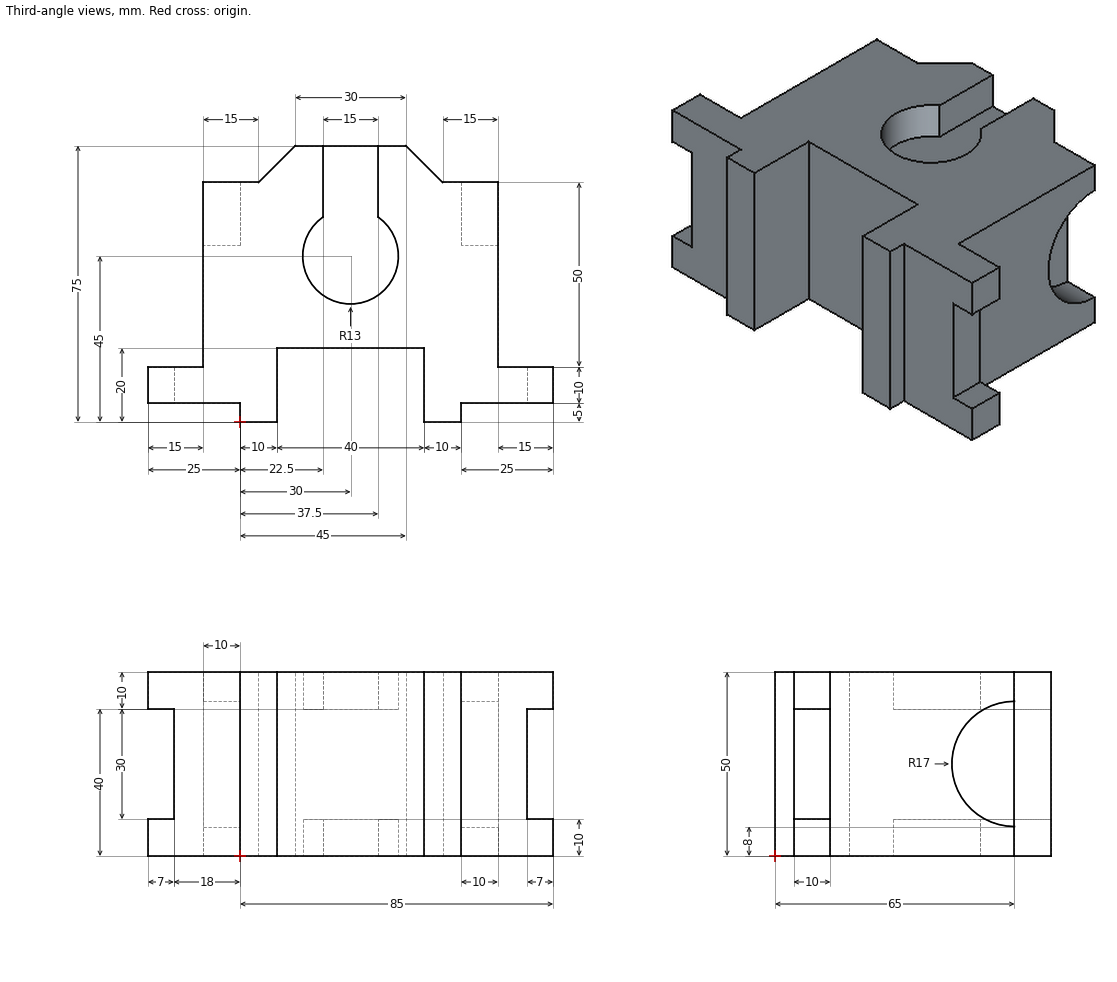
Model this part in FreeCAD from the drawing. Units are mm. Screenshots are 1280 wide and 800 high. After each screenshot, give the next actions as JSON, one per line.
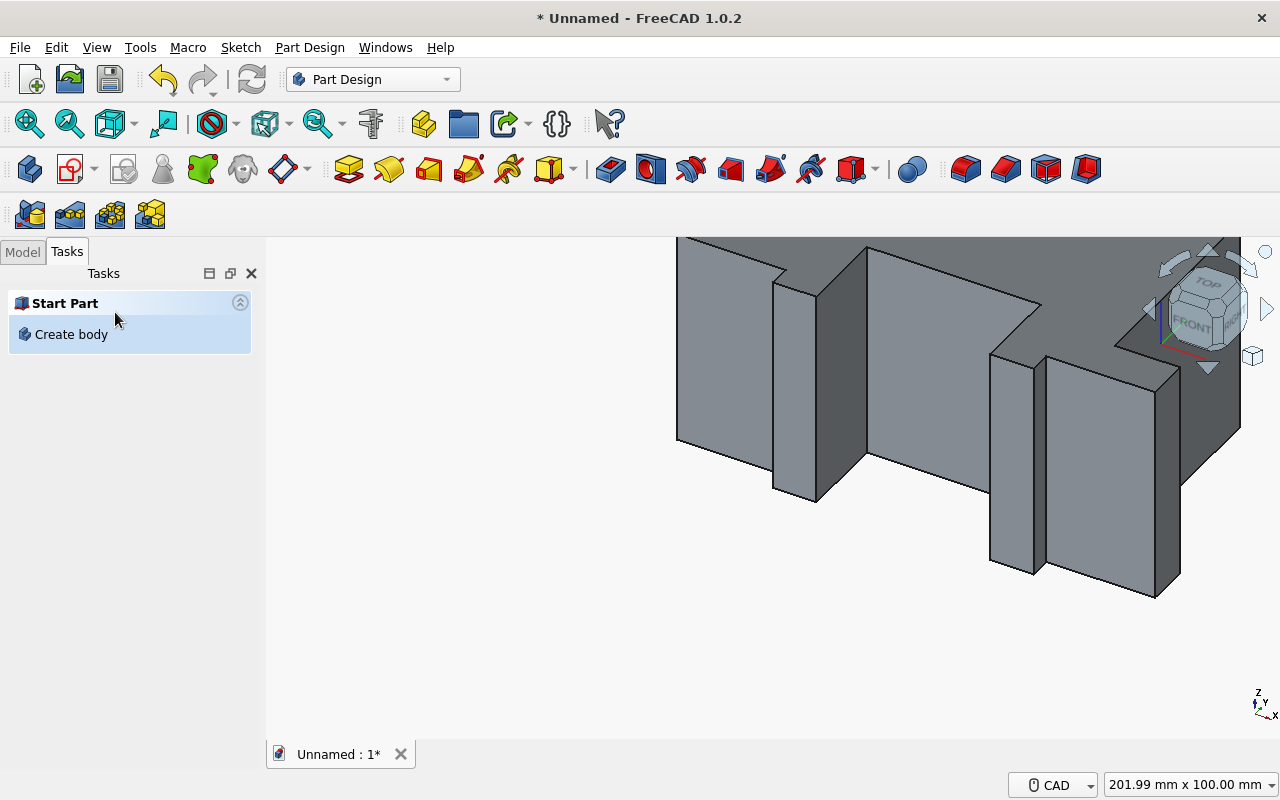
{"action": "left_click", "coordinate": [30, 124]}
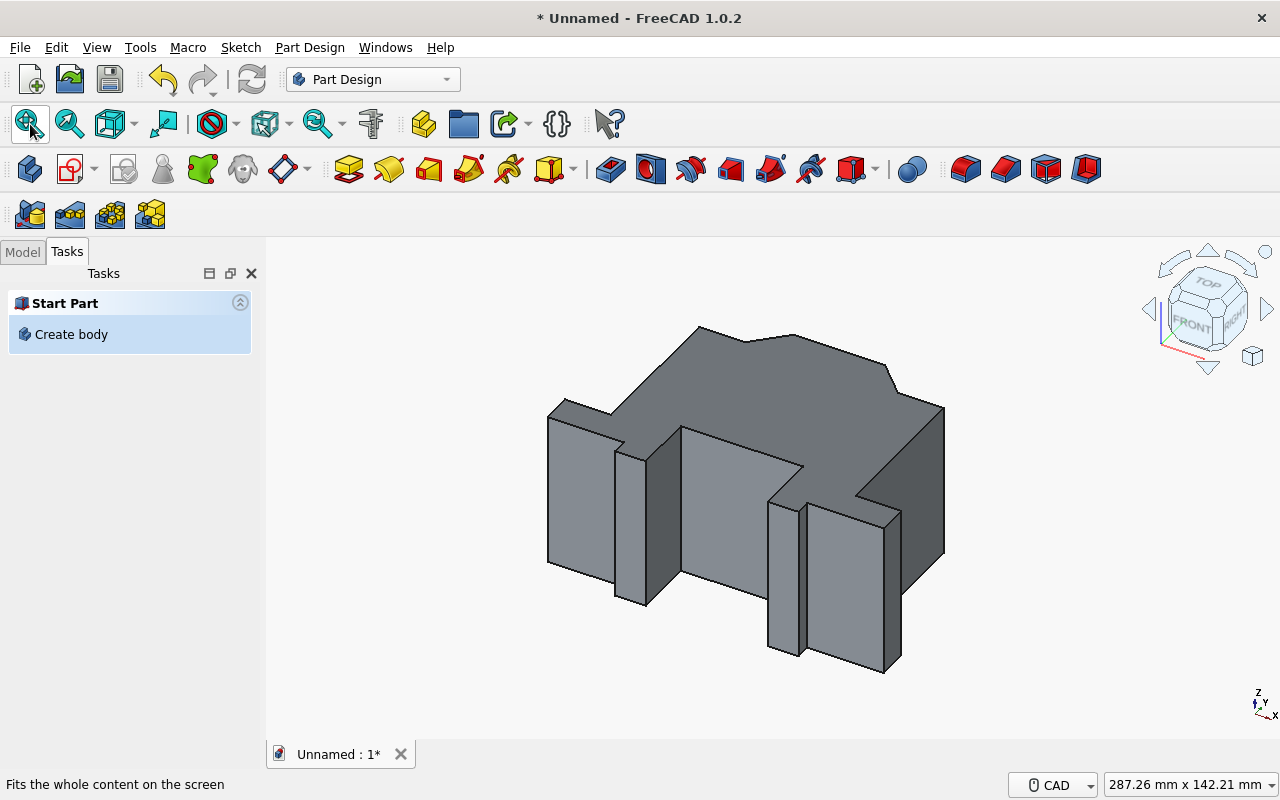
{"action": "key", "text": "6"}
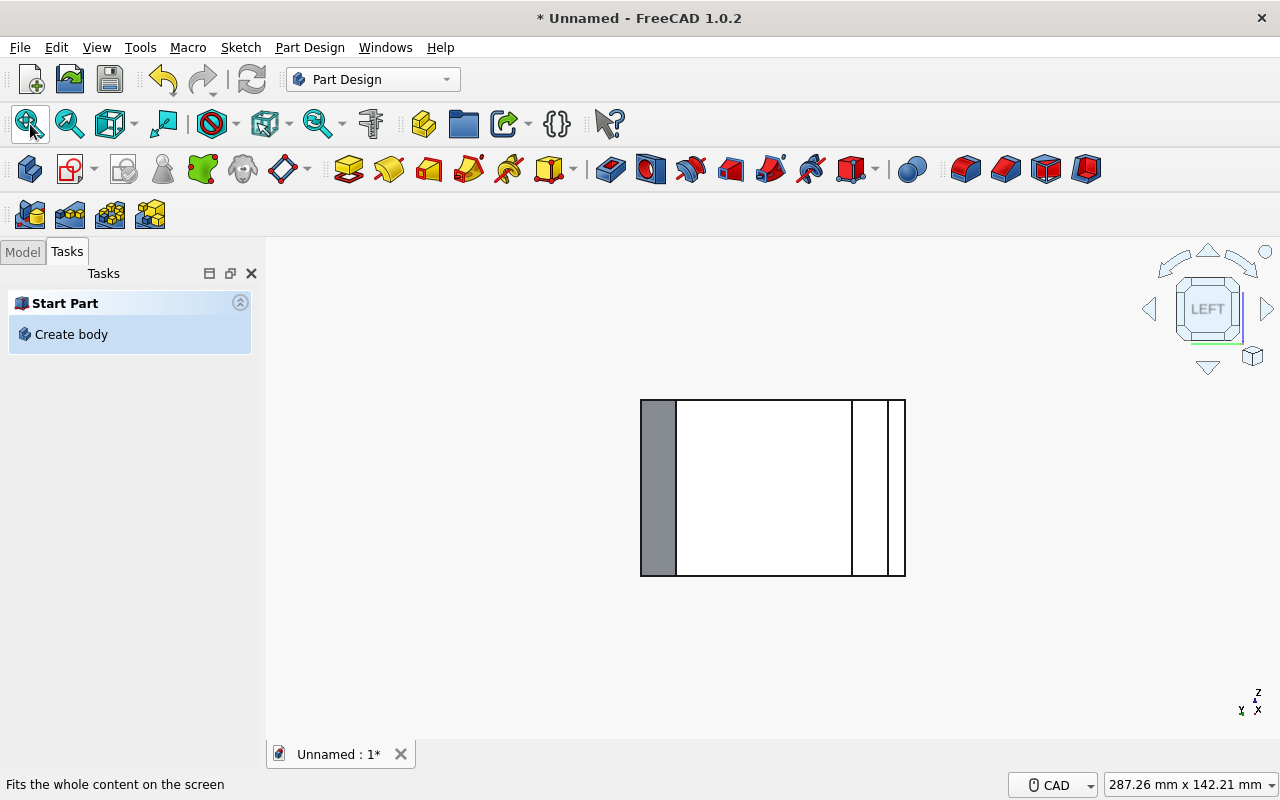
{"action": "key", "text": "v f"}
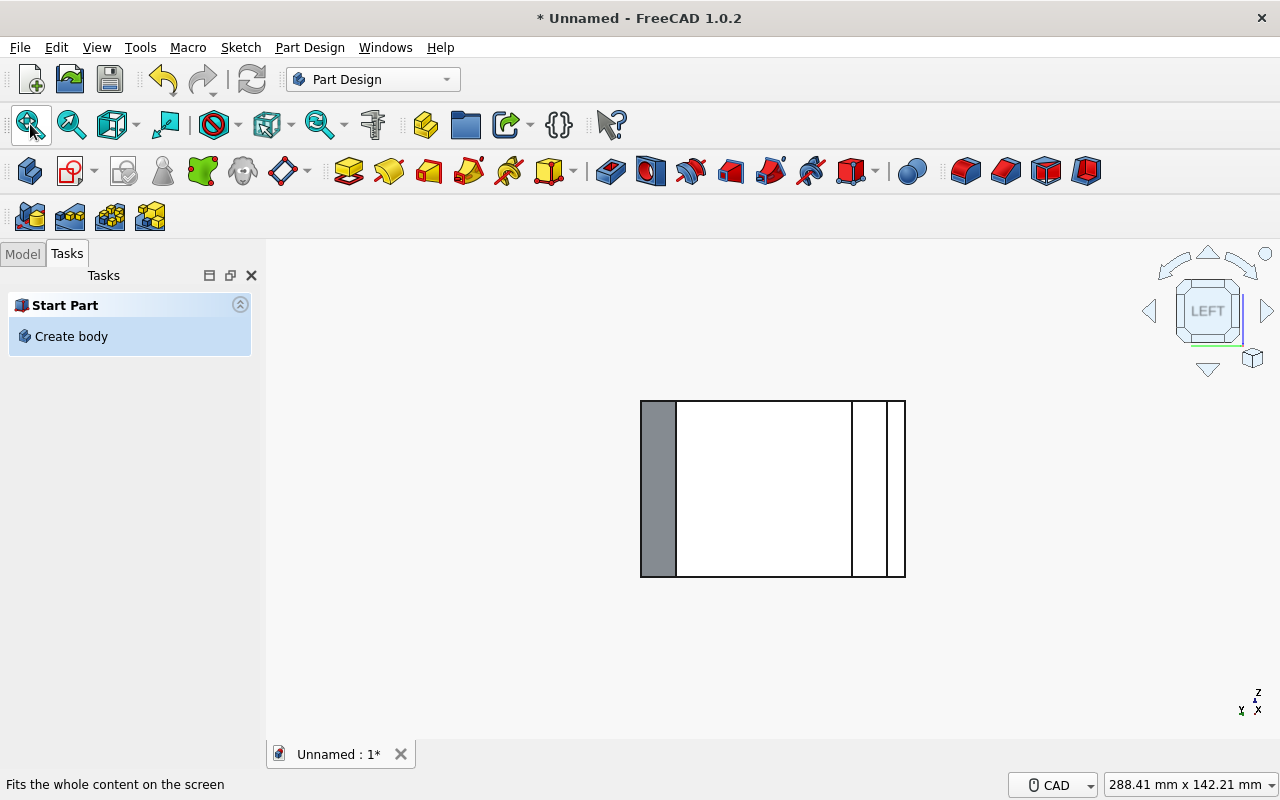
{"action": "left_click", "coordinate": [764, 488]}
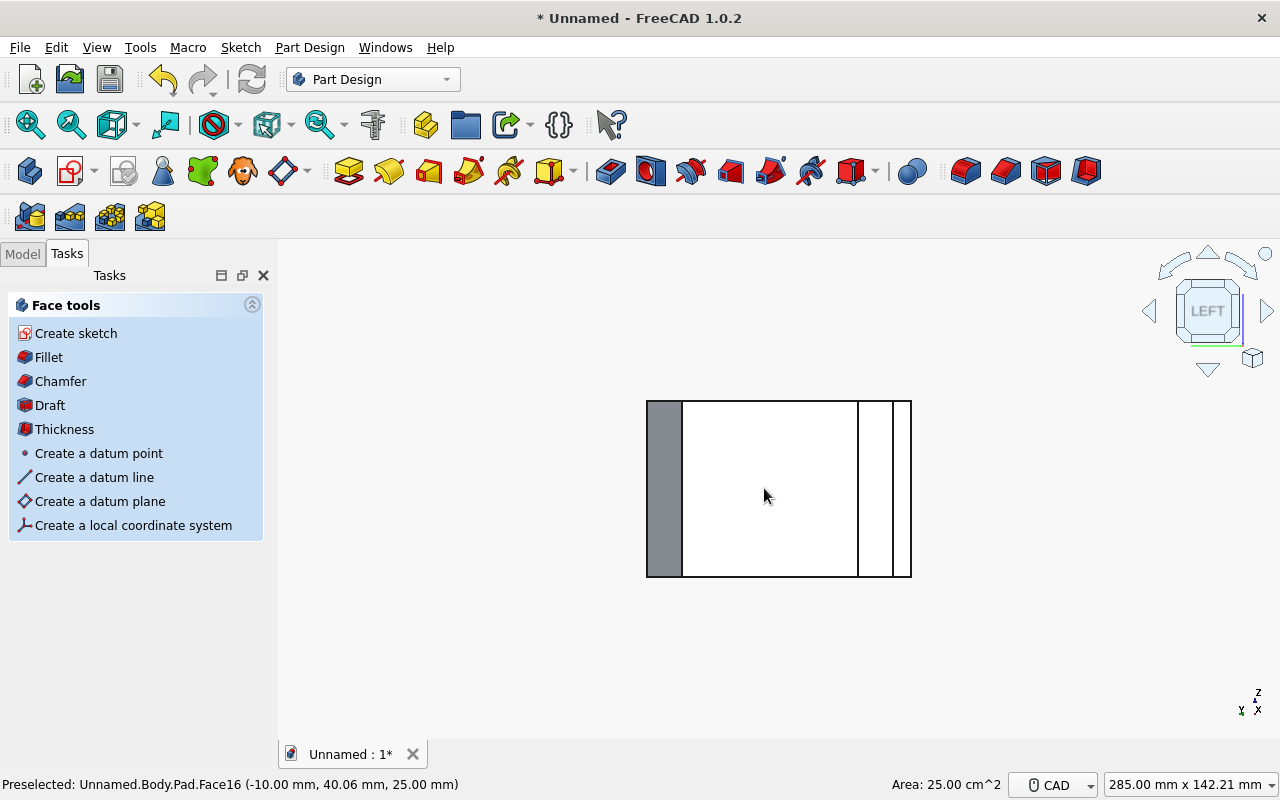
{"action": "left_click", "coordinate": [70, 172]}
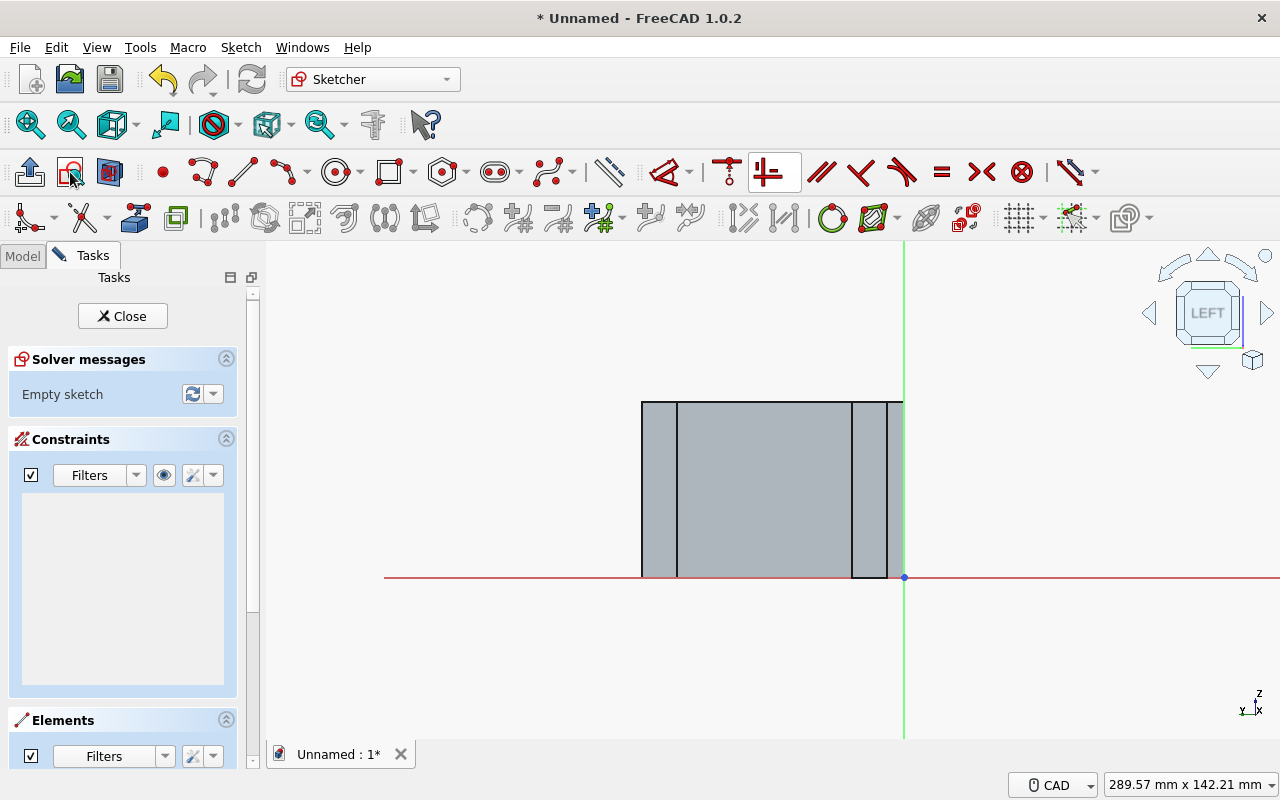
{"action": "left_click", "coordinate": [110, 172]}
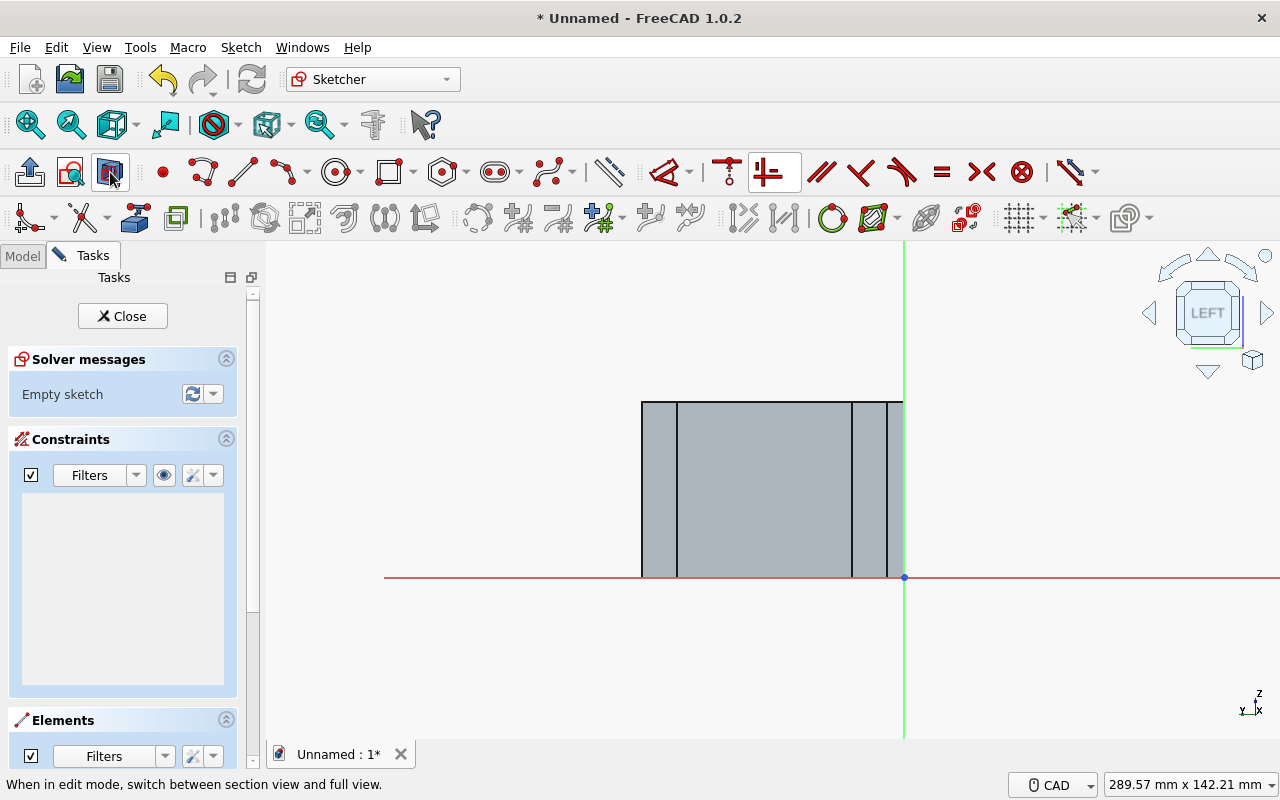
{"action": "scroll", "coordinate": [861, 515], "scroll_direction": "up", "scroll_amount": 4}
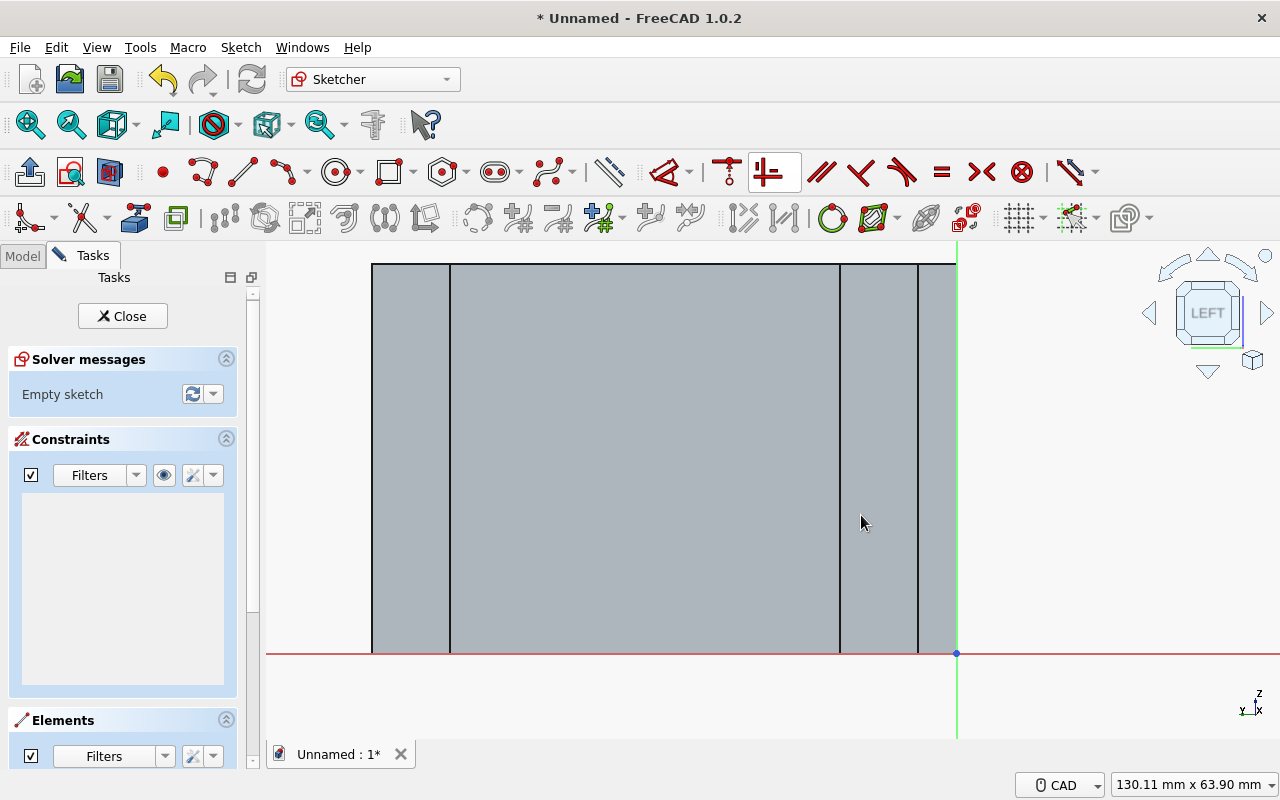
{"action": "key", "text": "g l"}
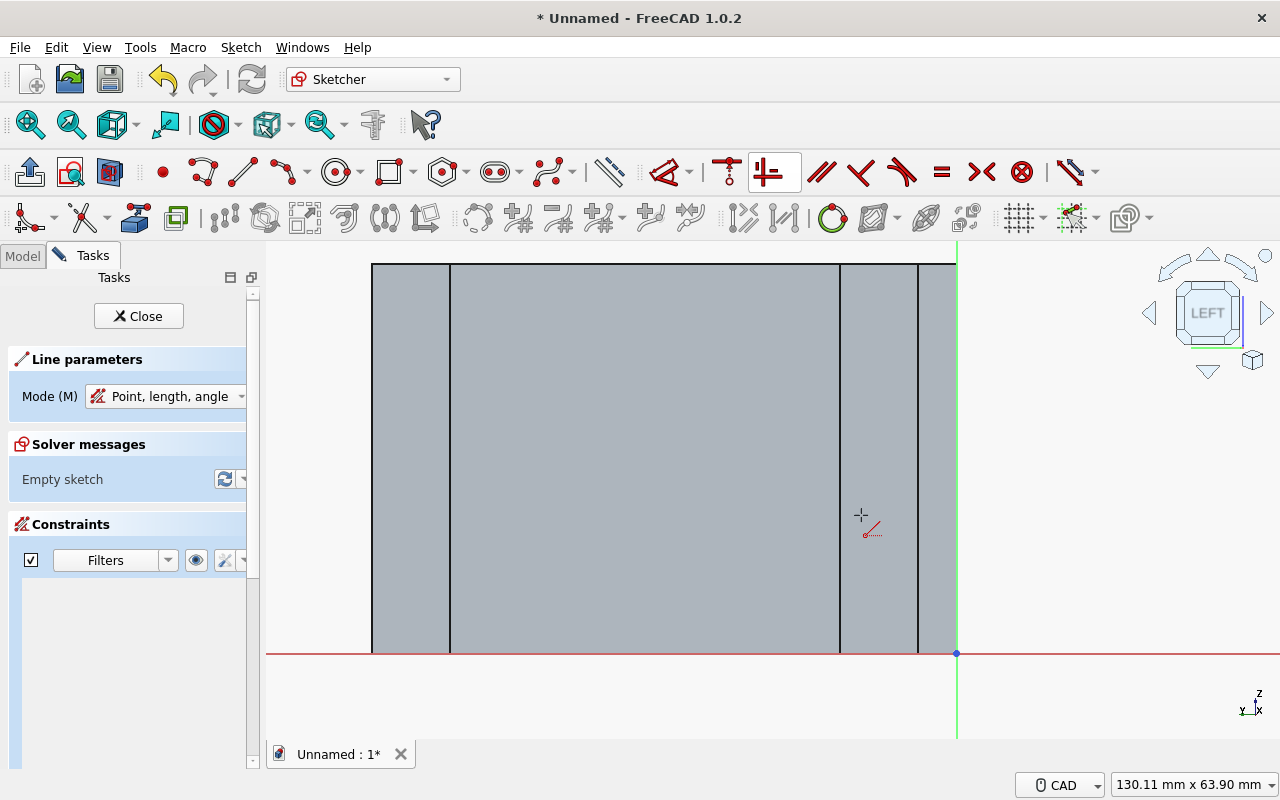
{"action": "left_click", "coordinate": [450, 326]}
{"action": "left_click", "coordinate": [450, 591]}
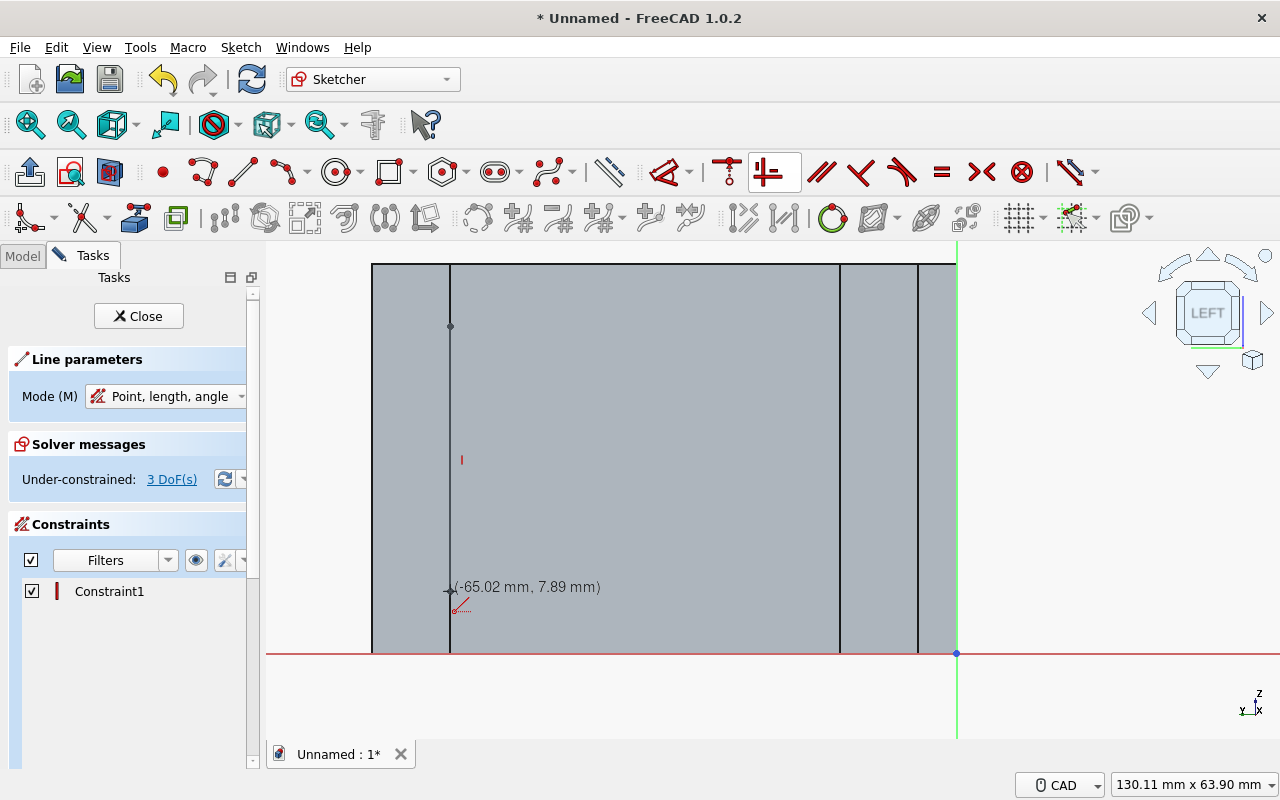
{"action": "key", "text": "g 3 a"}